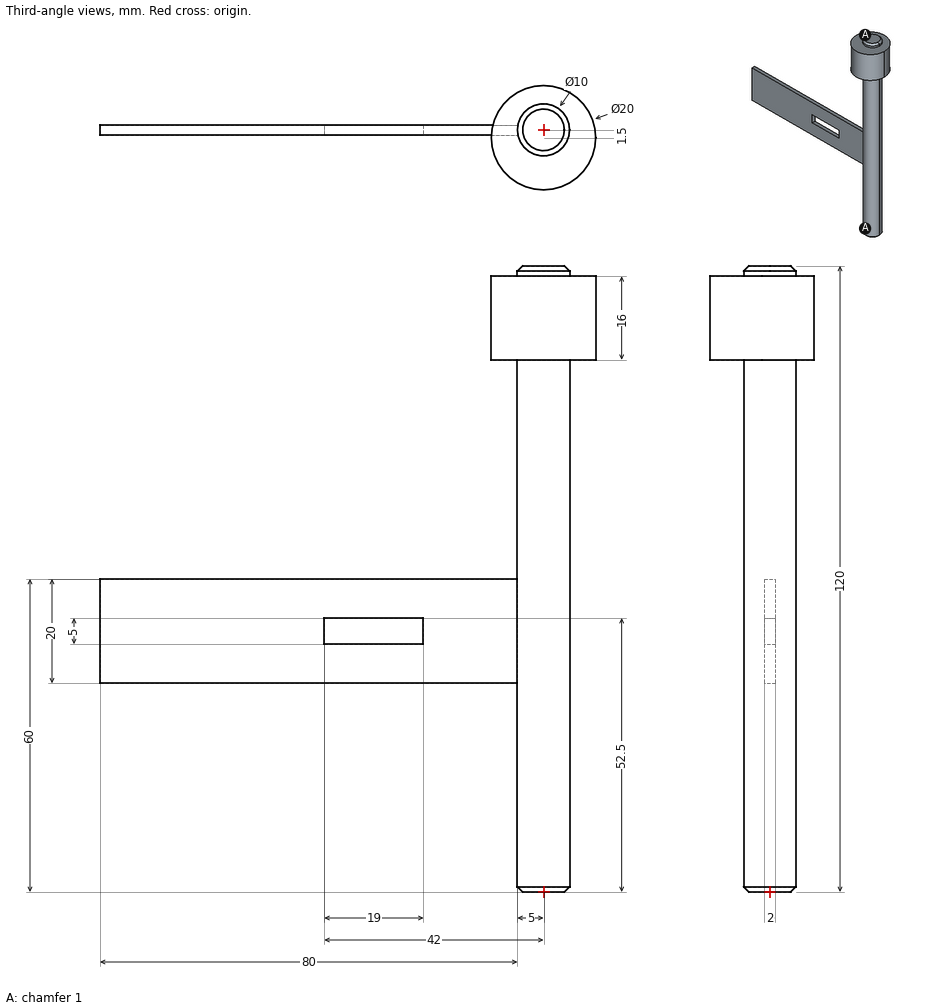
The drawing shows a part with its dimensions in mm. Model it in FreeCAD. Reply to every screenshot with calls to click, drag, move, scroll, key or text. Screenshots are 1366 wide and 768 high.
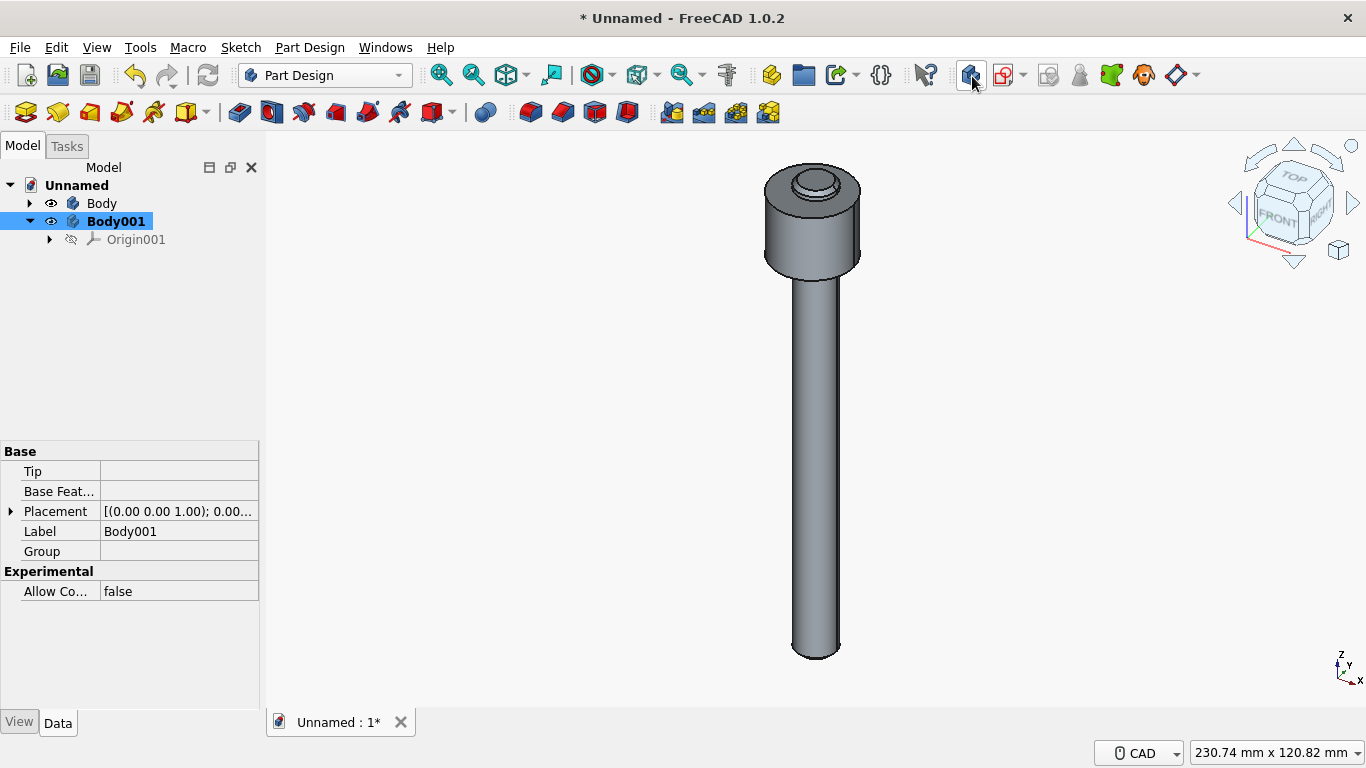
click(306, 667)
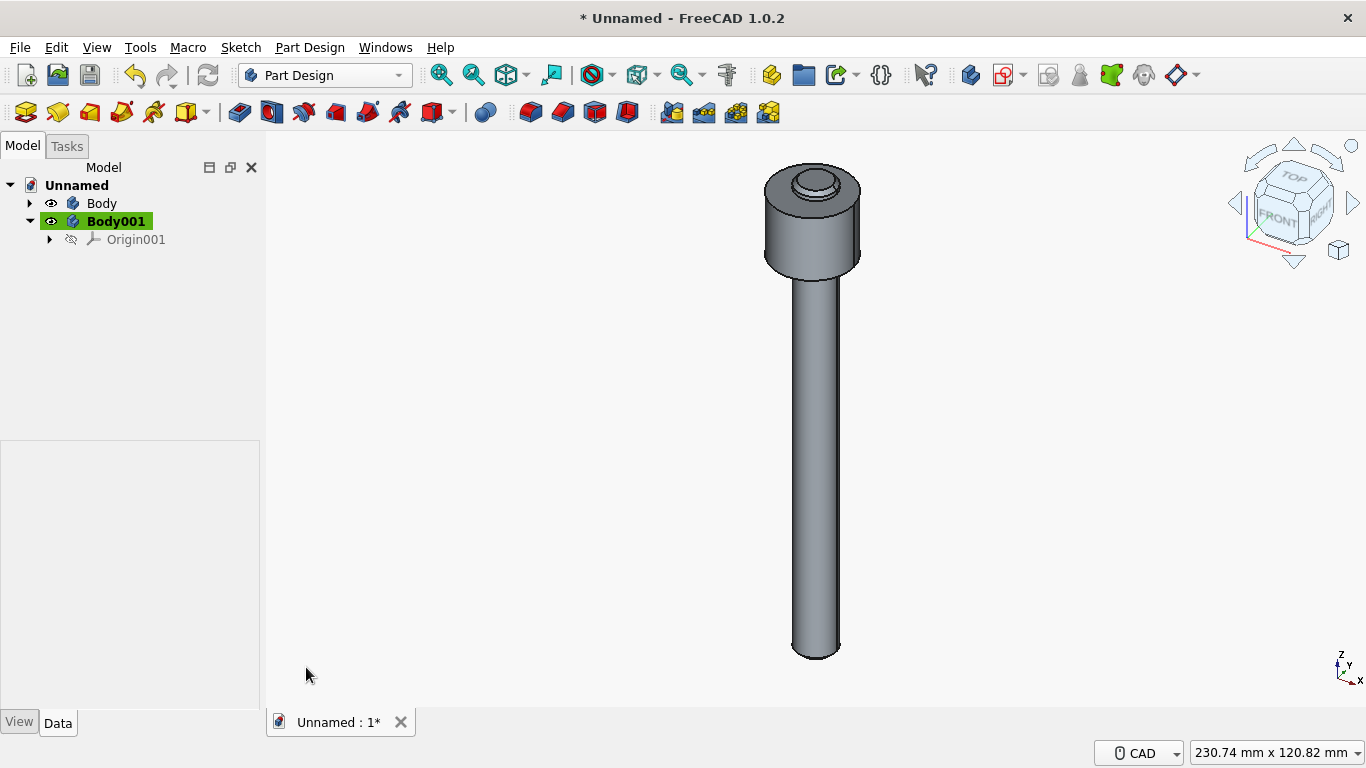
click(1004, 76)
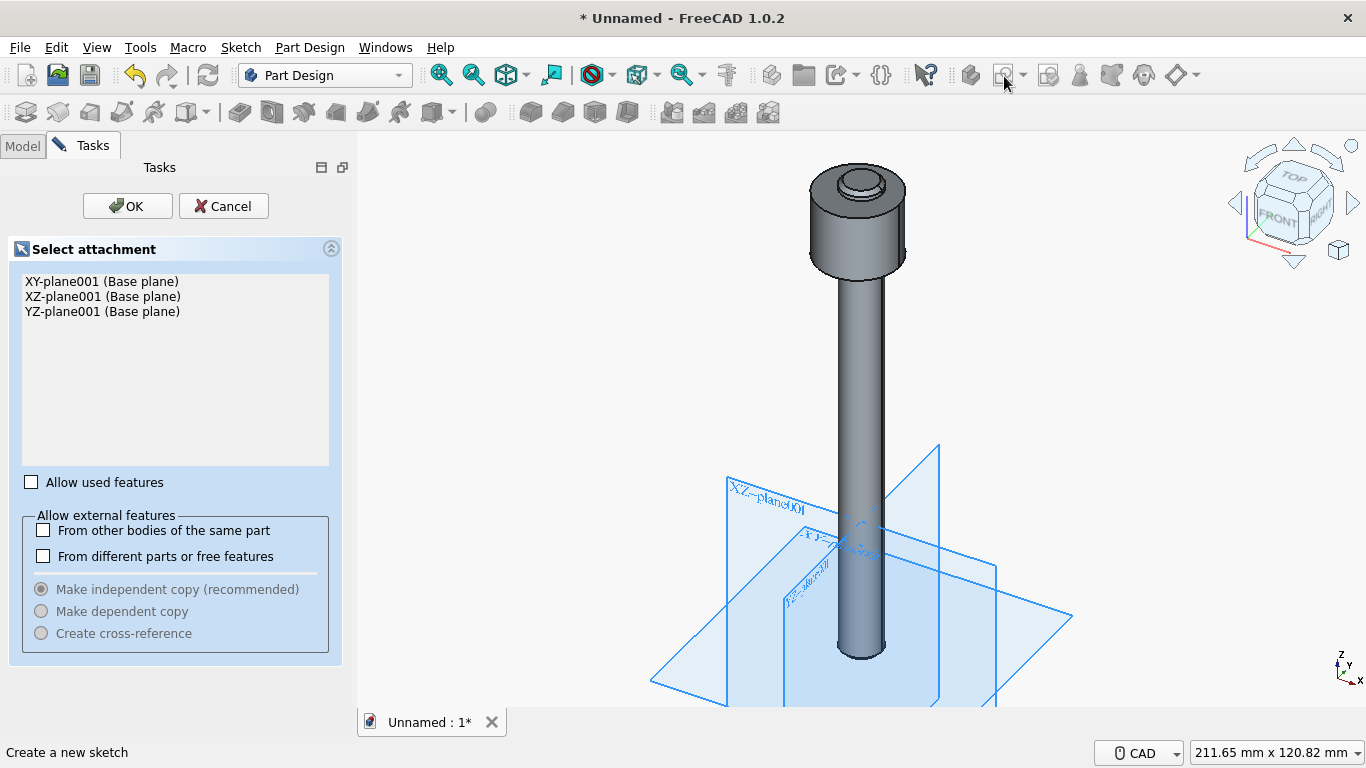
click(82, 296)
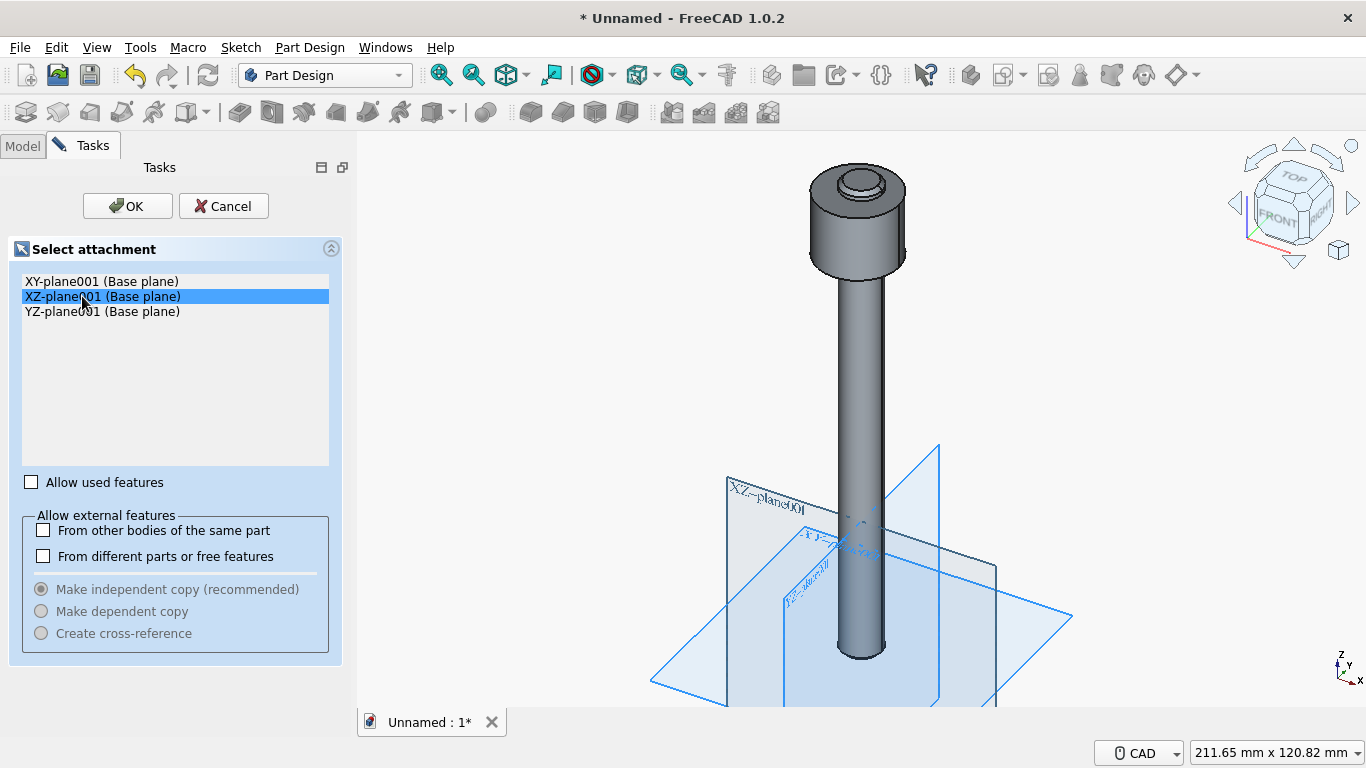
click(128, 206)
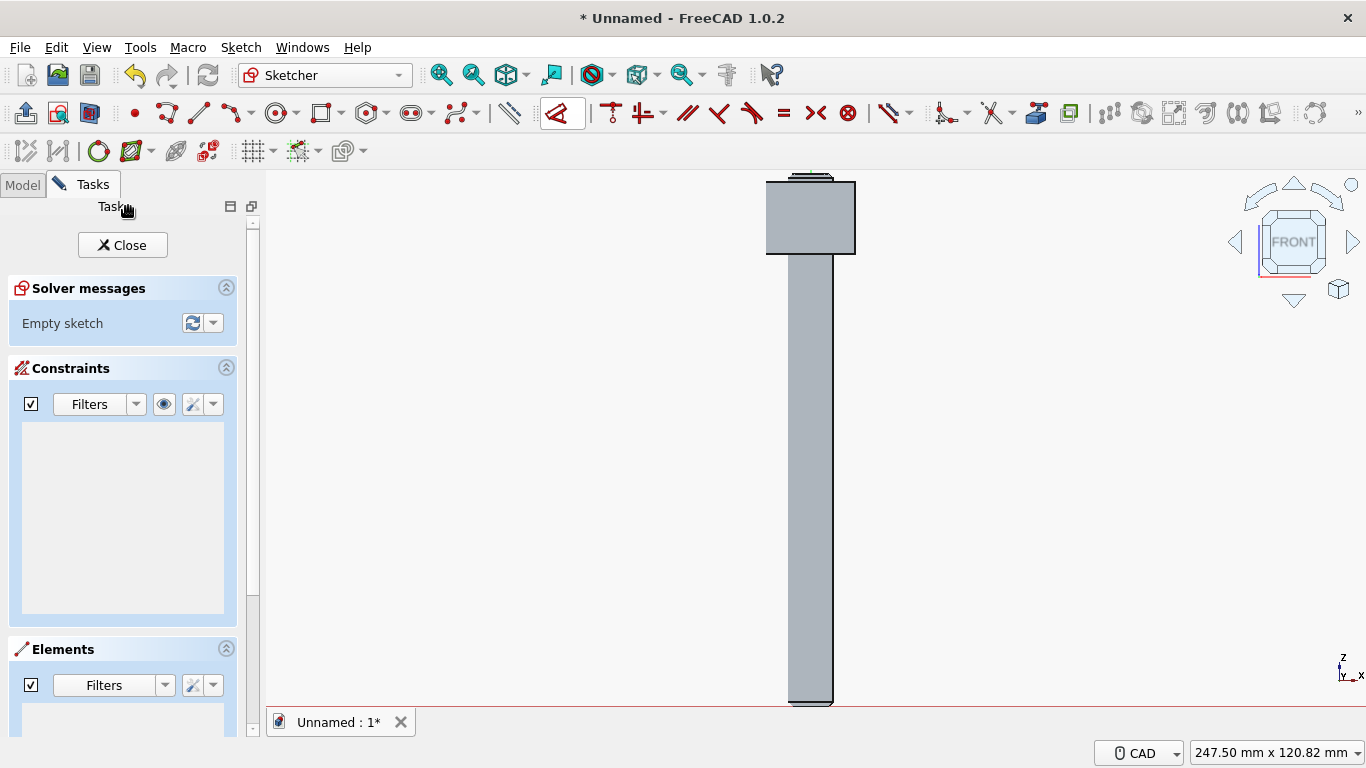
scroll(1201, 198, down, 1)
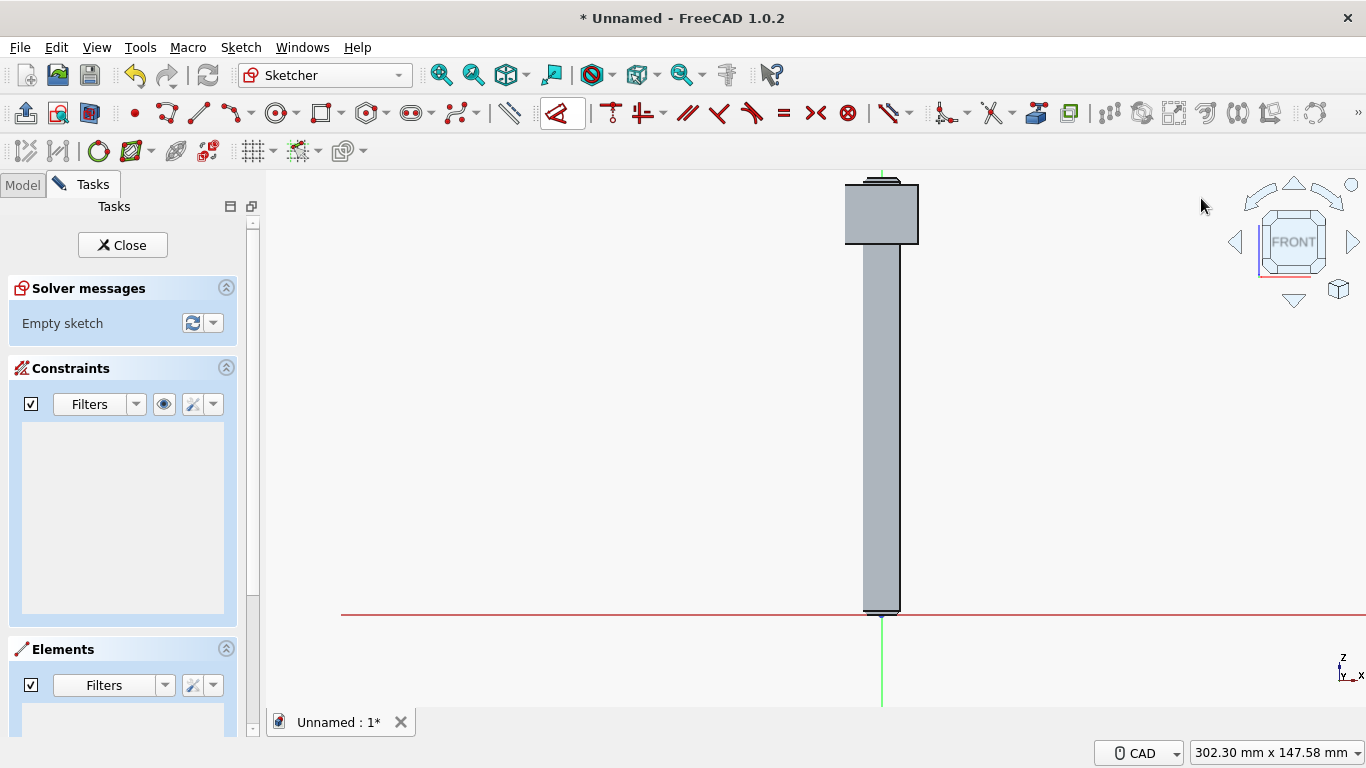
scroll(685, 642, up, 2)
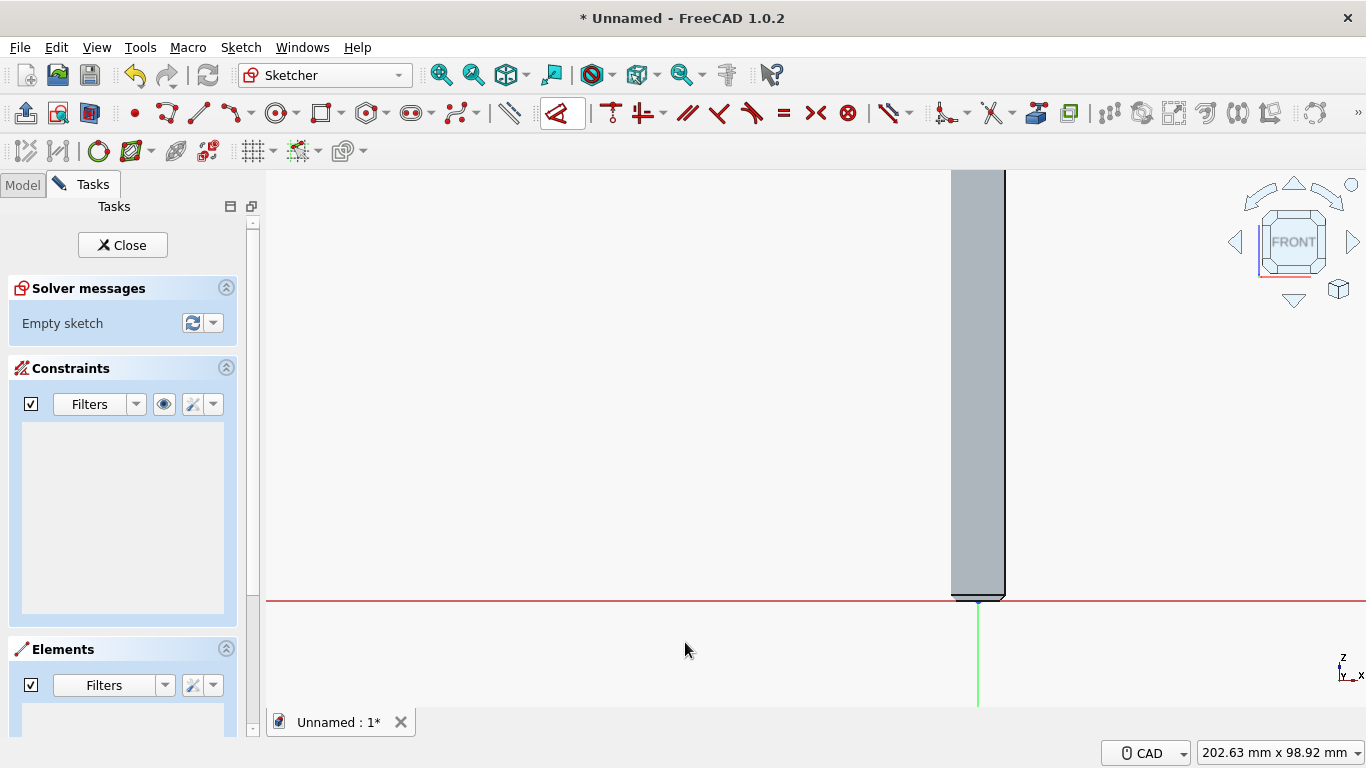
click(322, 114)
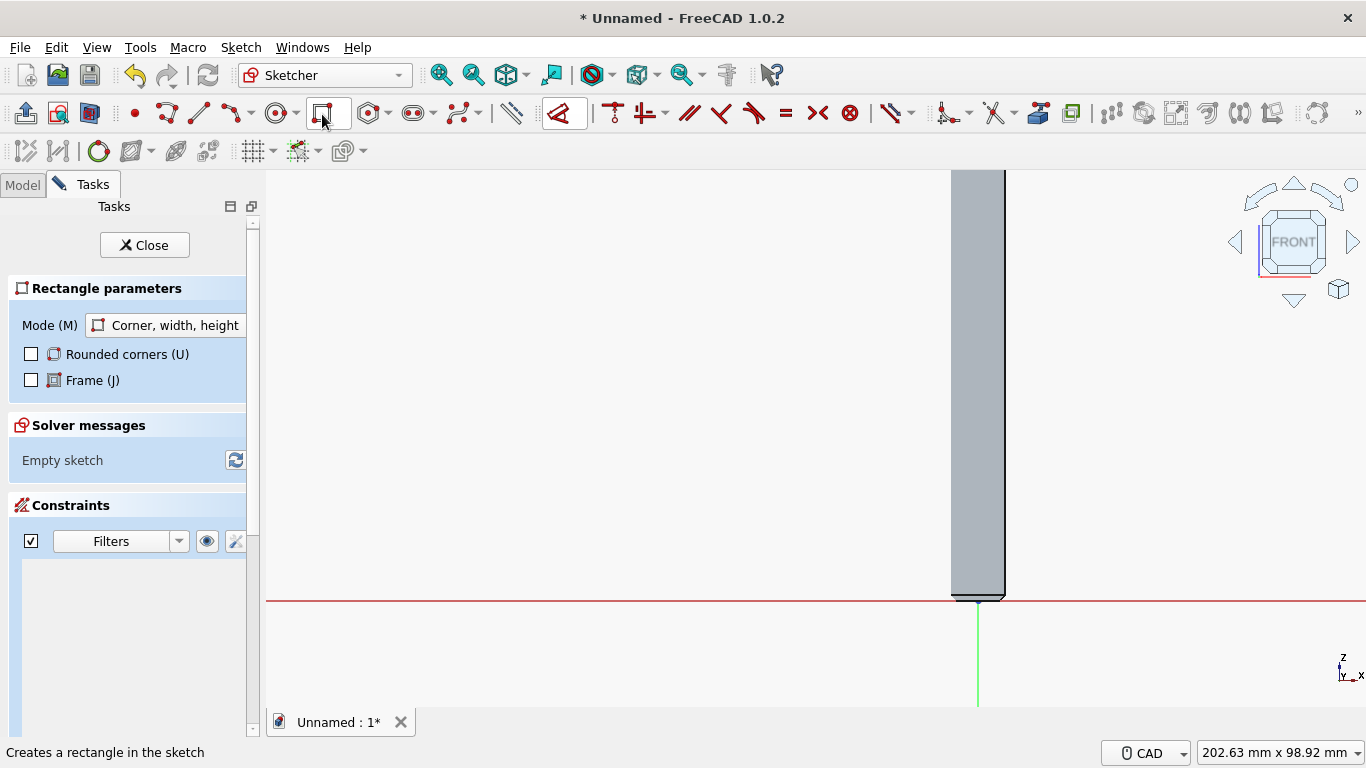
click(517, 275)
click(951, 384)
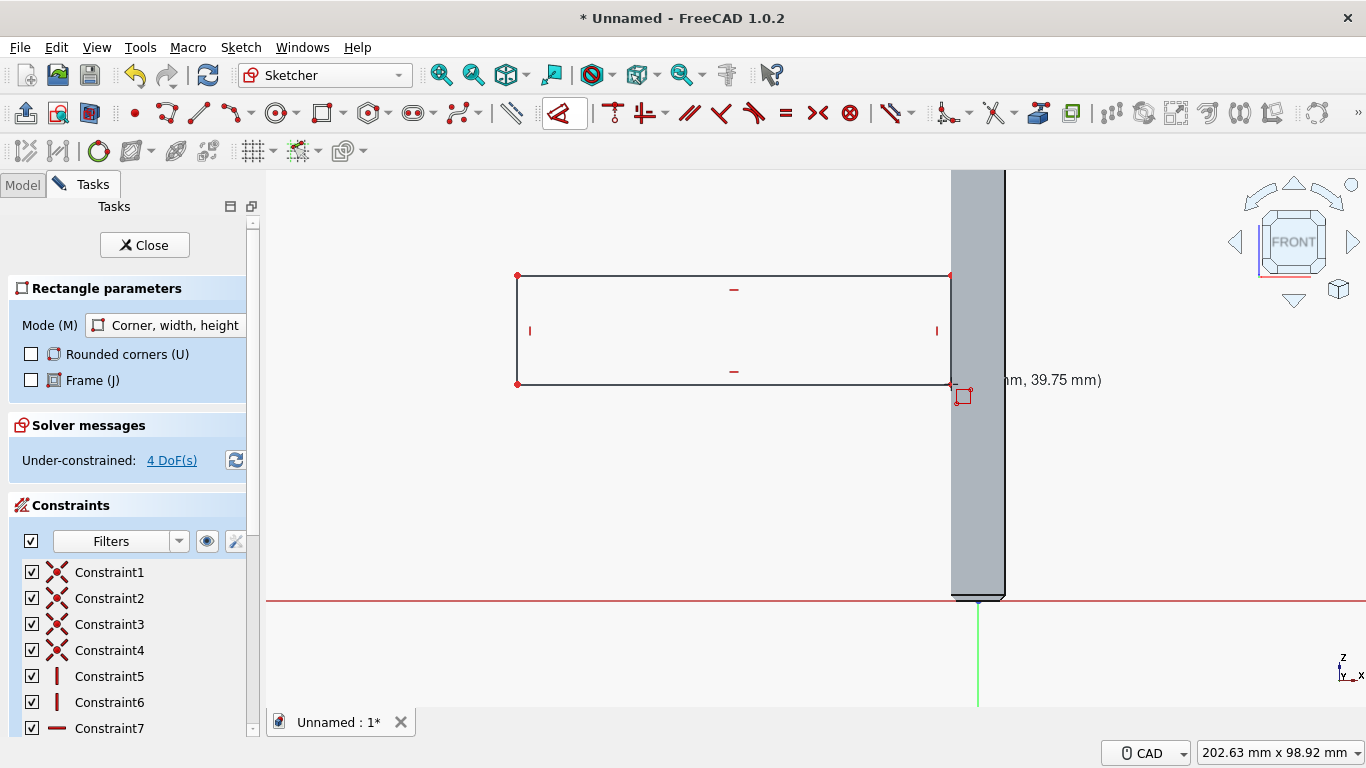
click(750, 316)
click(853, 343)
key(Escape)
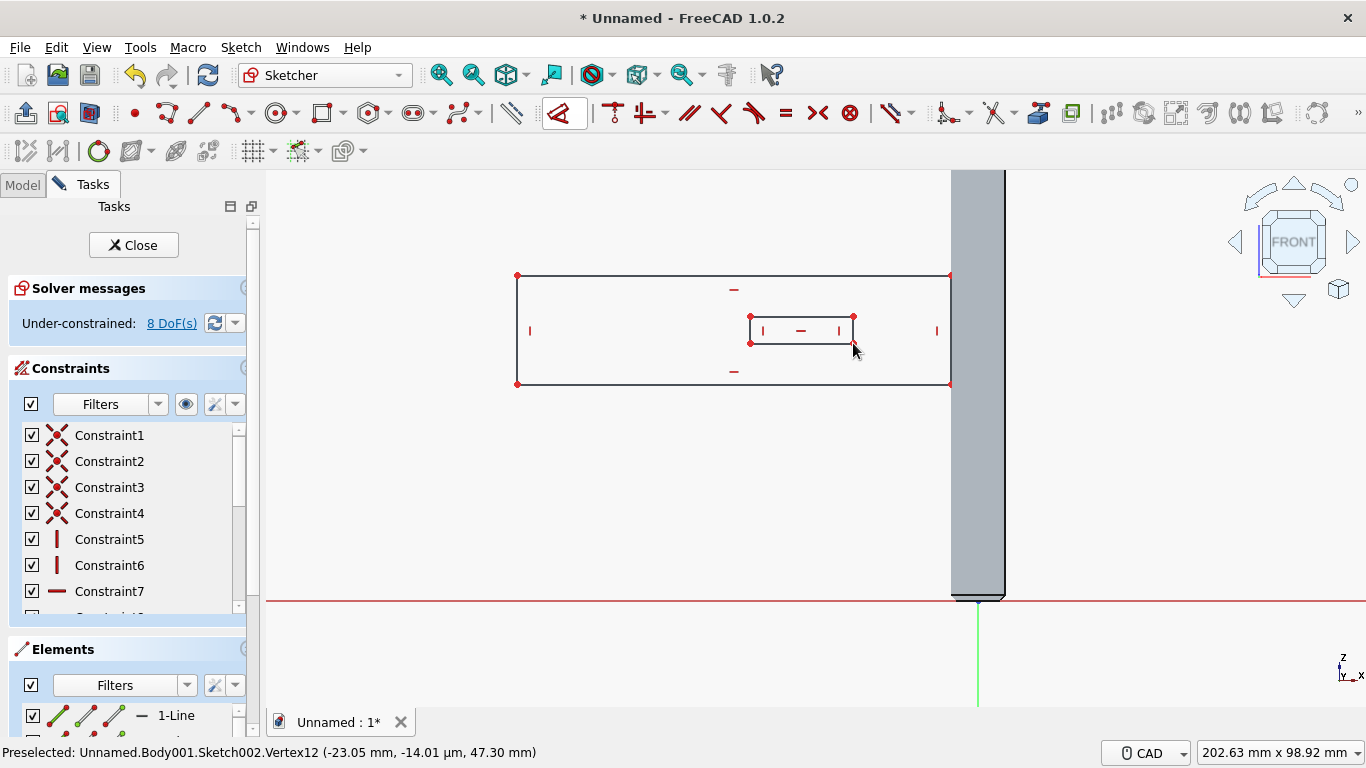
scroll(750, 328, up, 2)